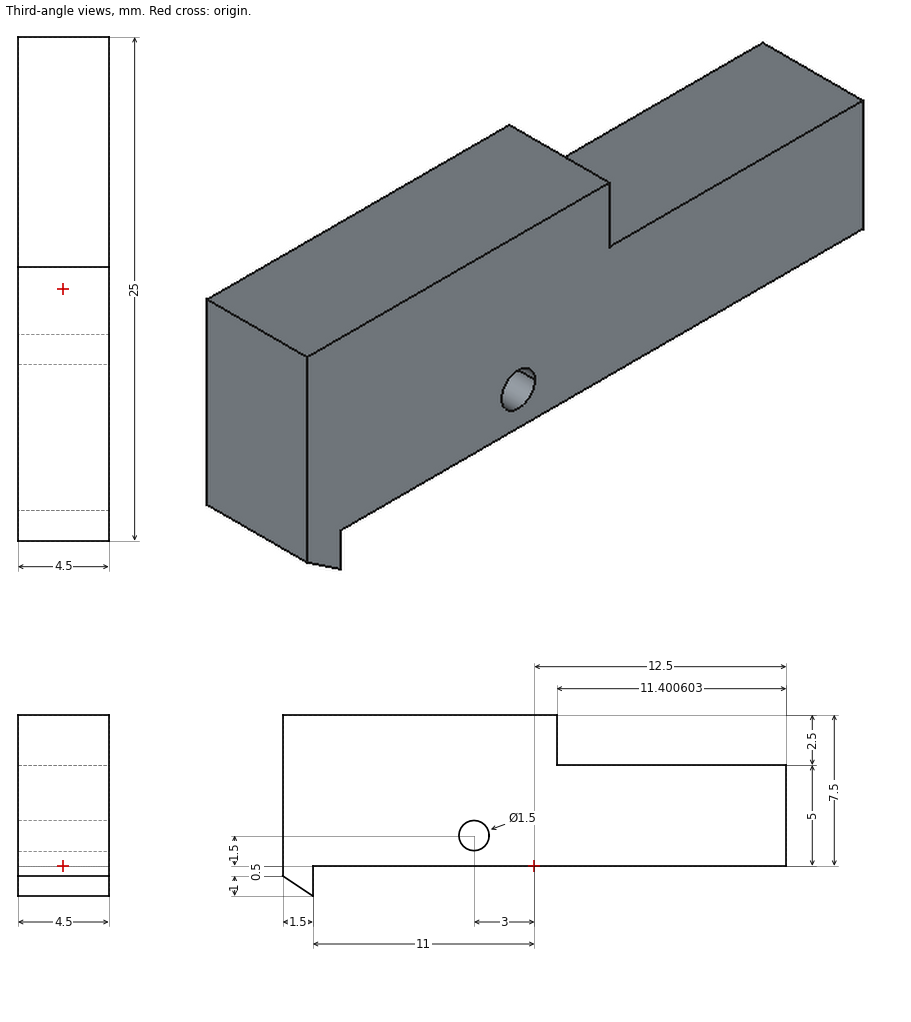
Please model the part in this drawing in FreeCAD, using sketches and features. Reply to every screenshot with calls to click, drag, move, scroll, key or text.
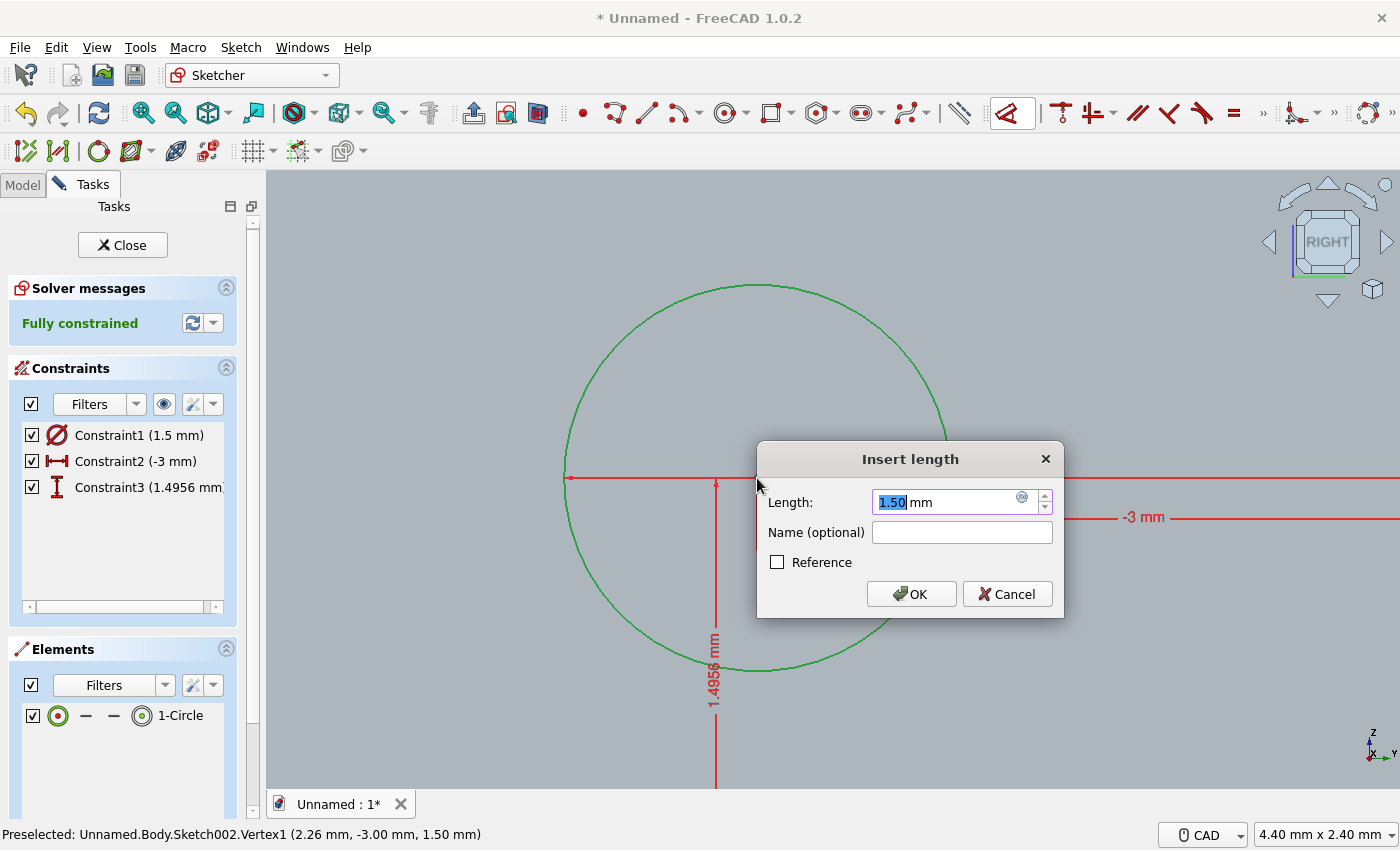
text(1.5)
key(Return)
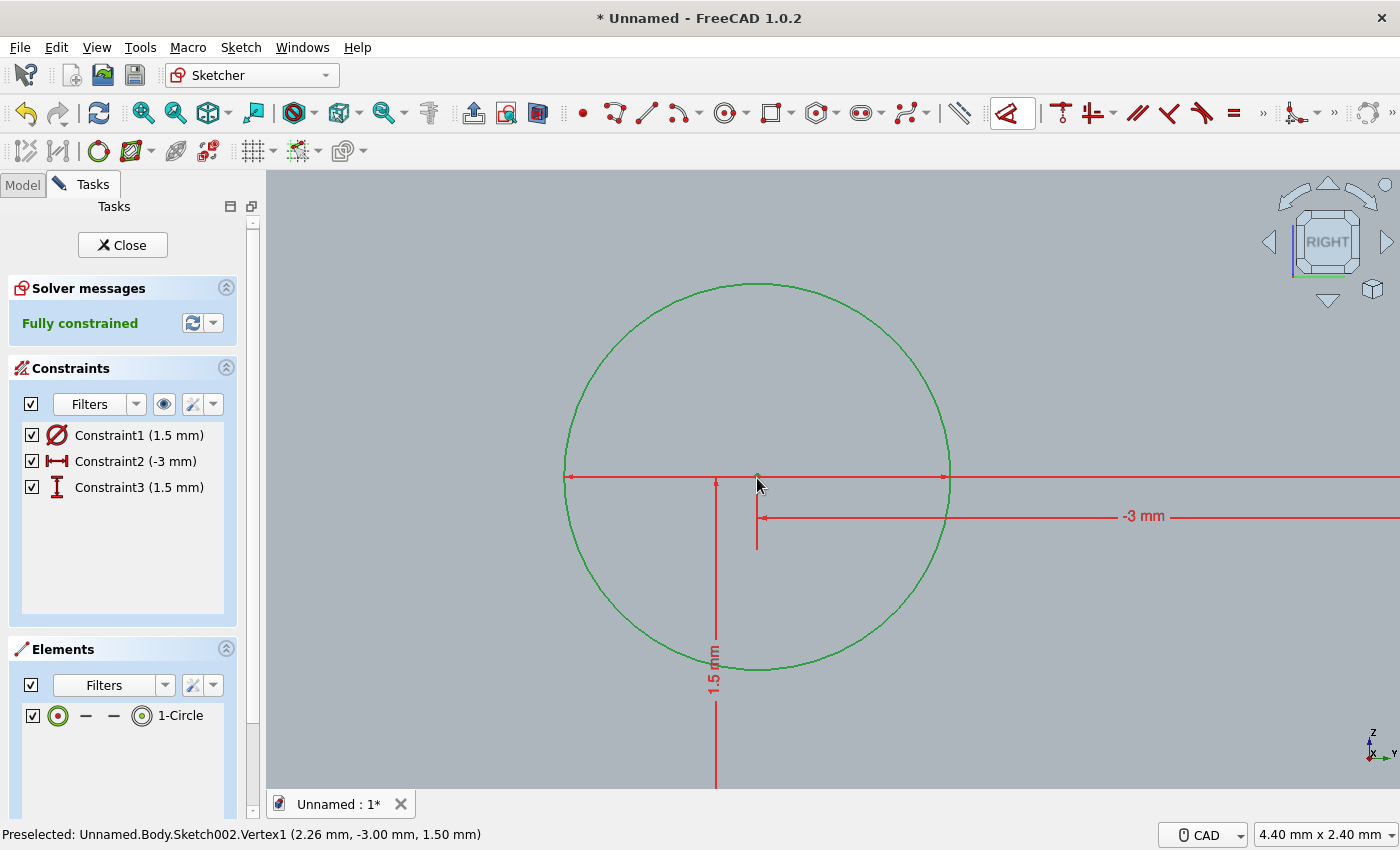
click(123, 245)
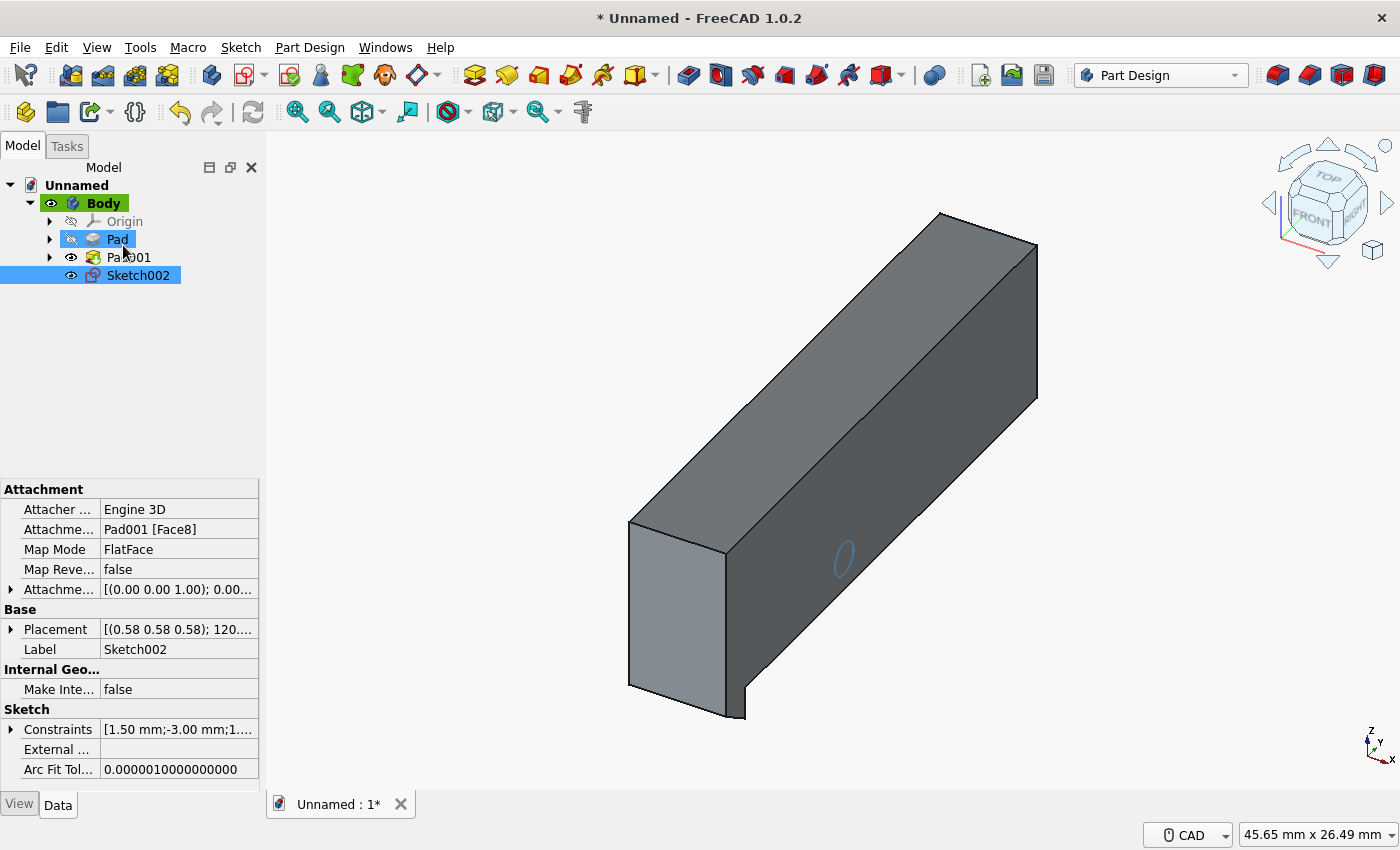
click(690, 76)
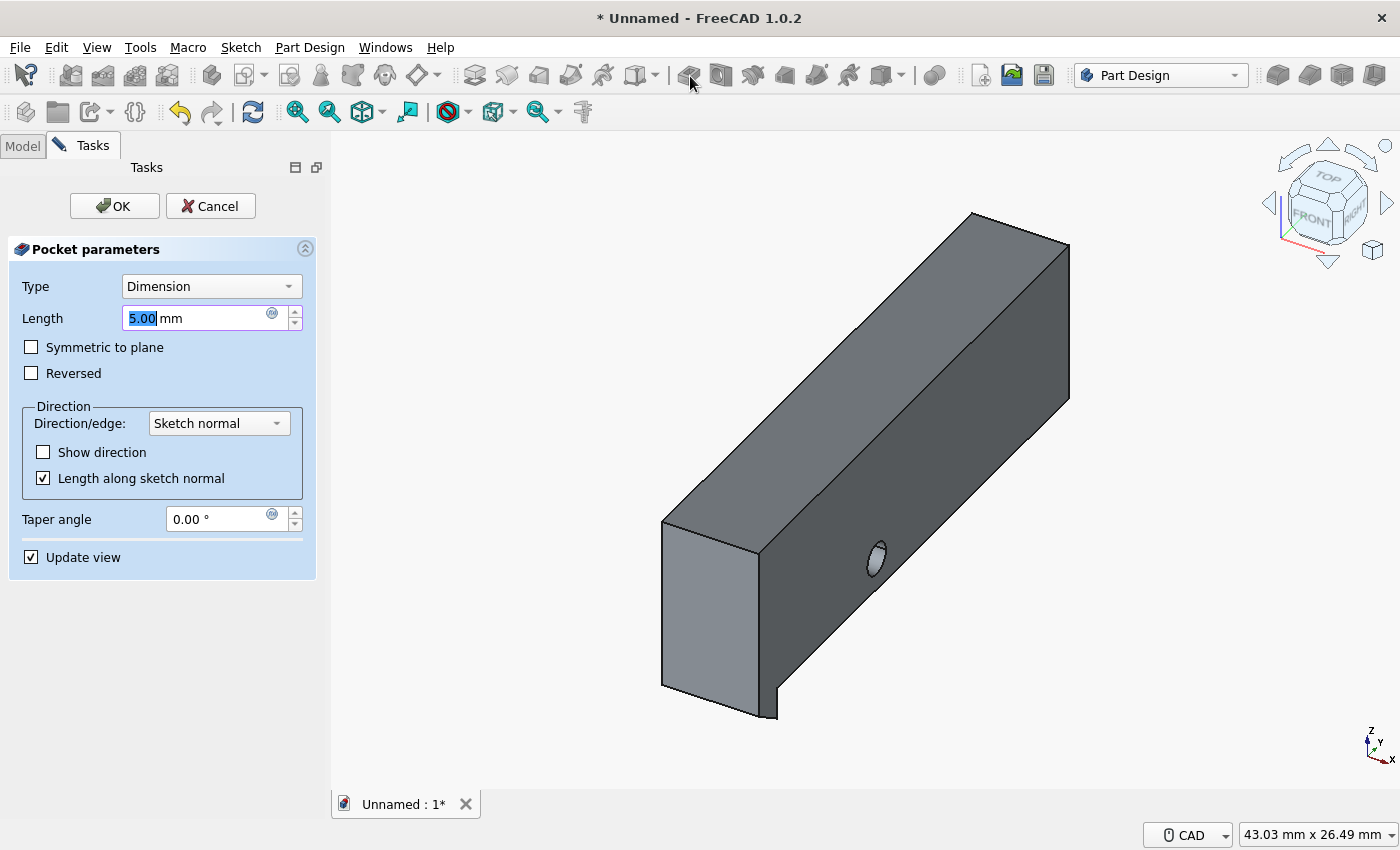
click(212, 286)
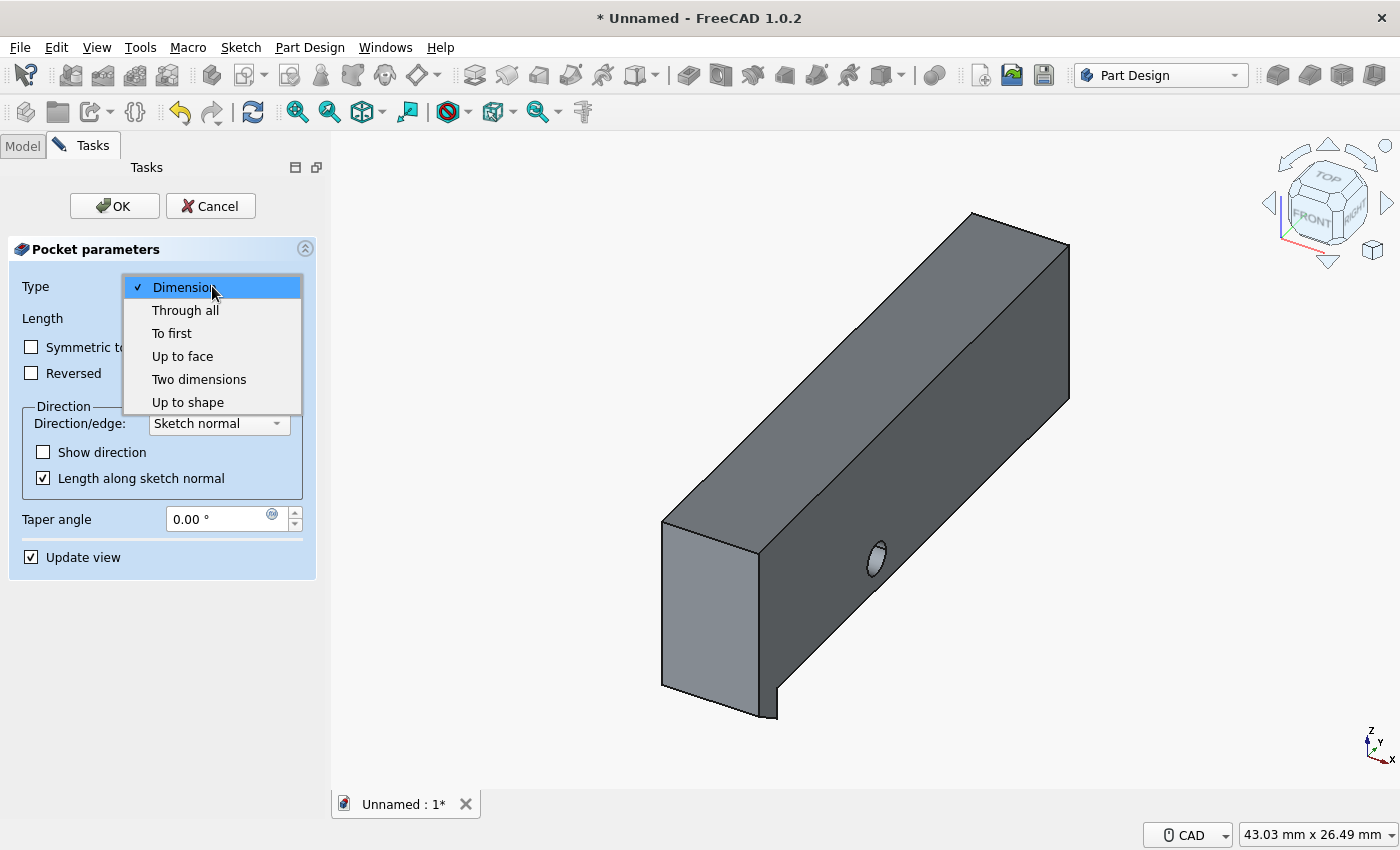
click(212, 310)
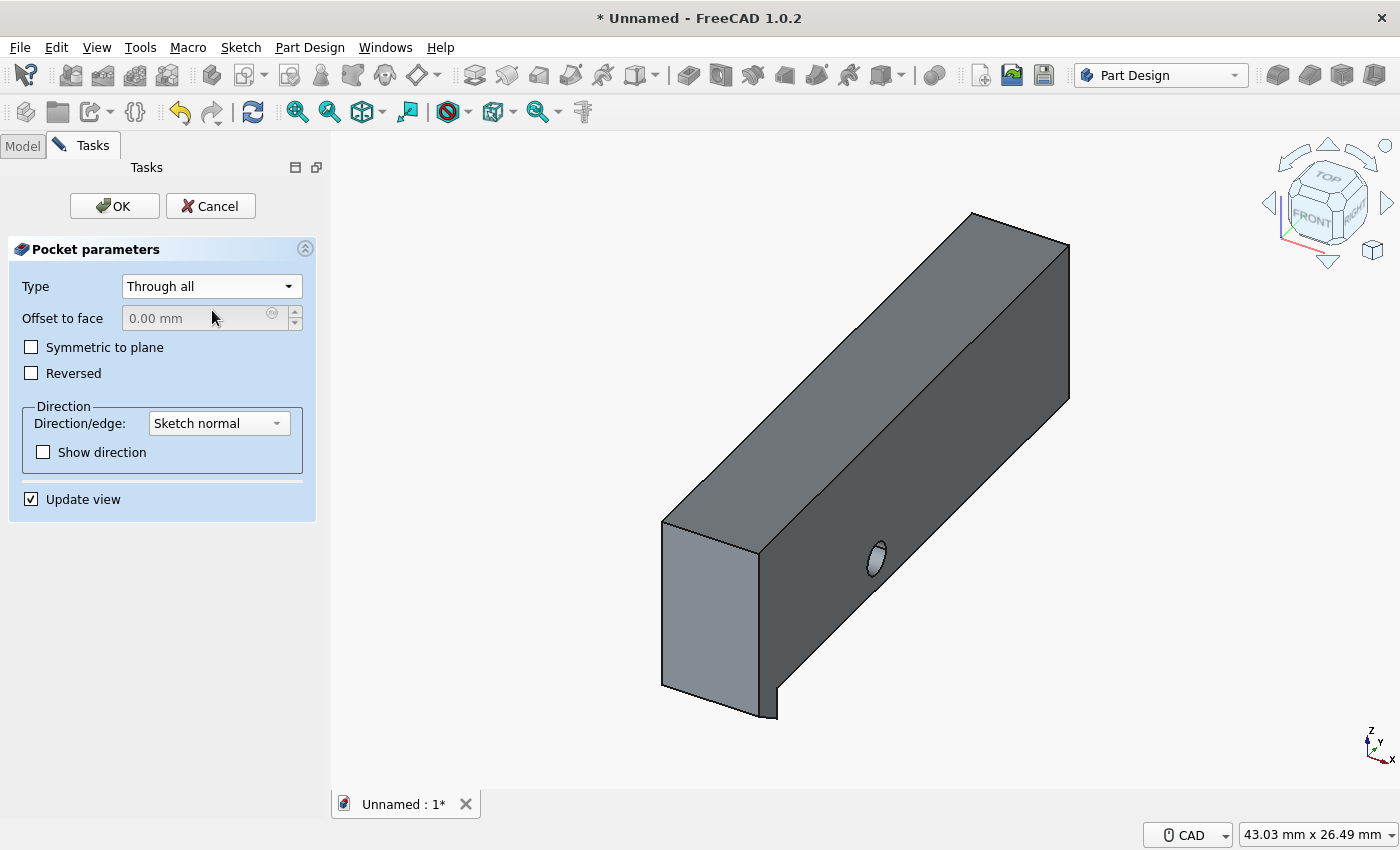
click(115, 206)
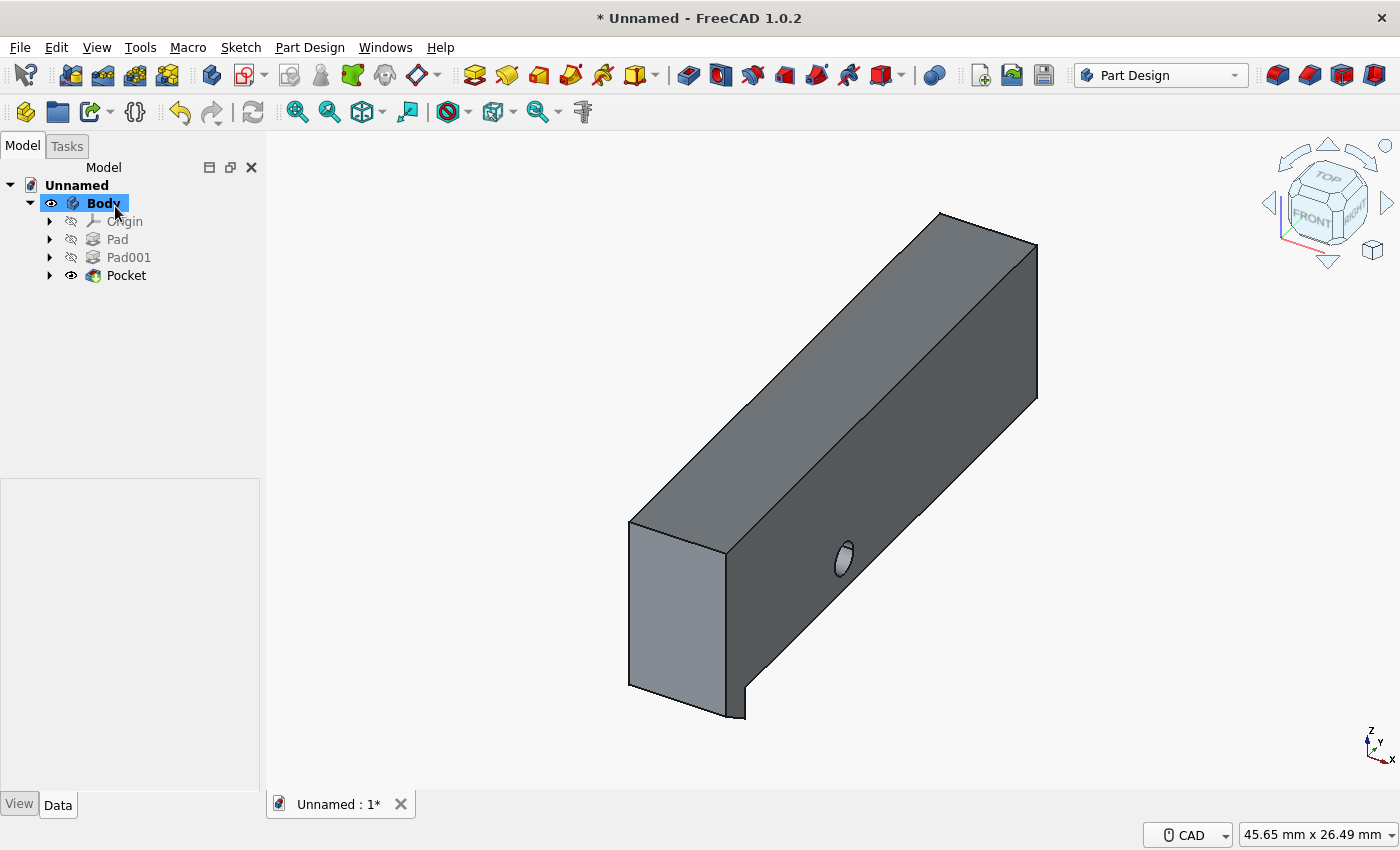
key(6)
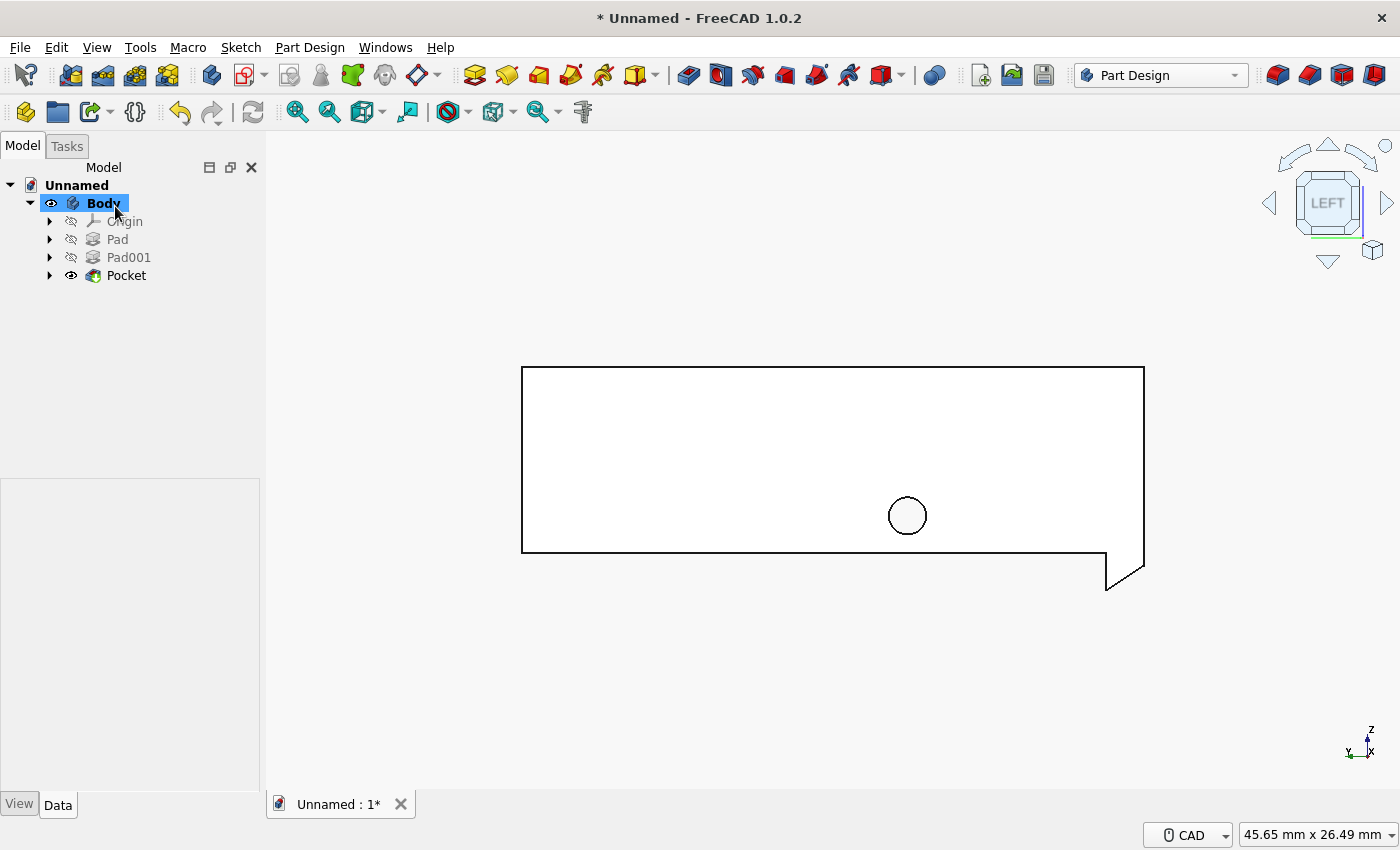
click(656, 446)